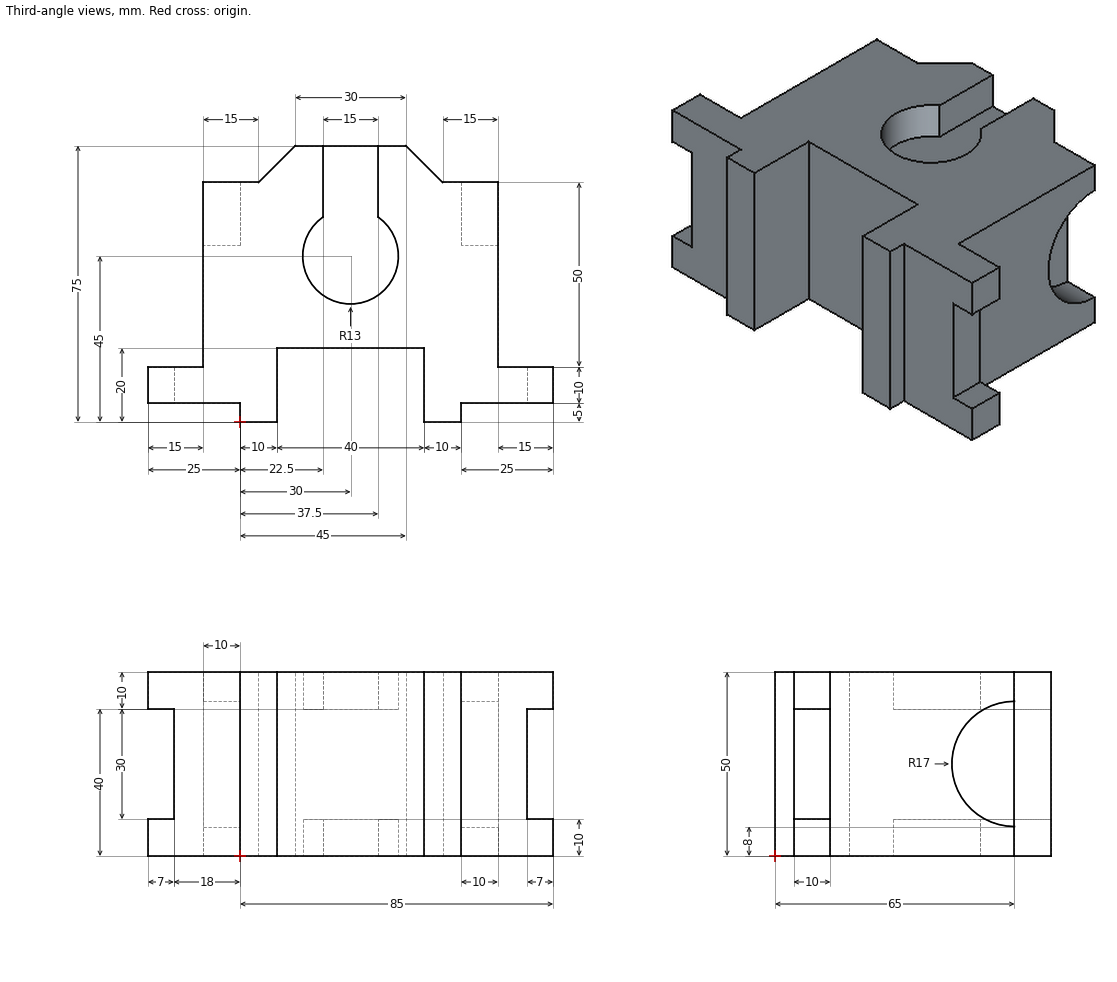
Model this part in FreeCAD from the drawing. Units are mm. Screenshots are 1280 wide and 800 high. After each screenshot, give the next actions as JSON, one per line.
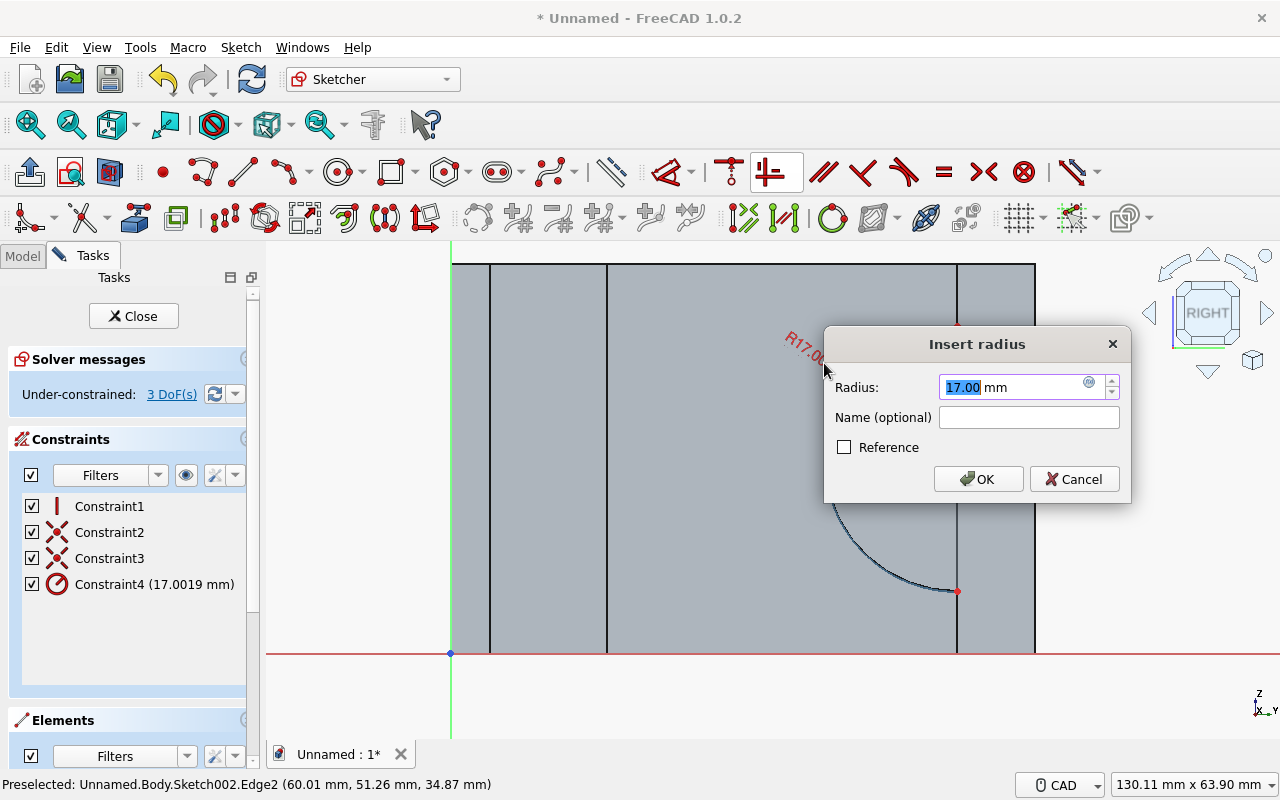
{"action": "type", "text": "17"}
{"action": "key", "text": "Return"}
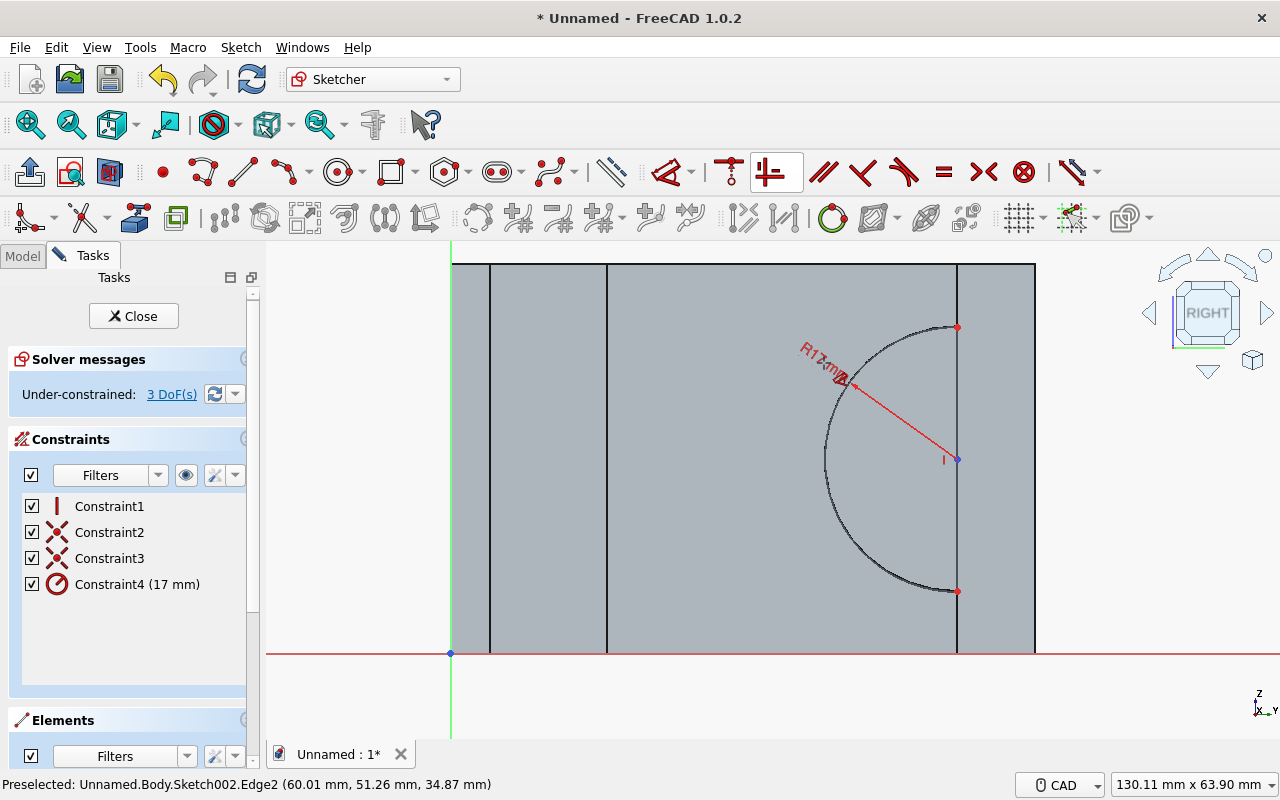
{"action": "left_click", "coordinate": [957, 592]}
{"action": "left_click", "coordinate": [417, 623]}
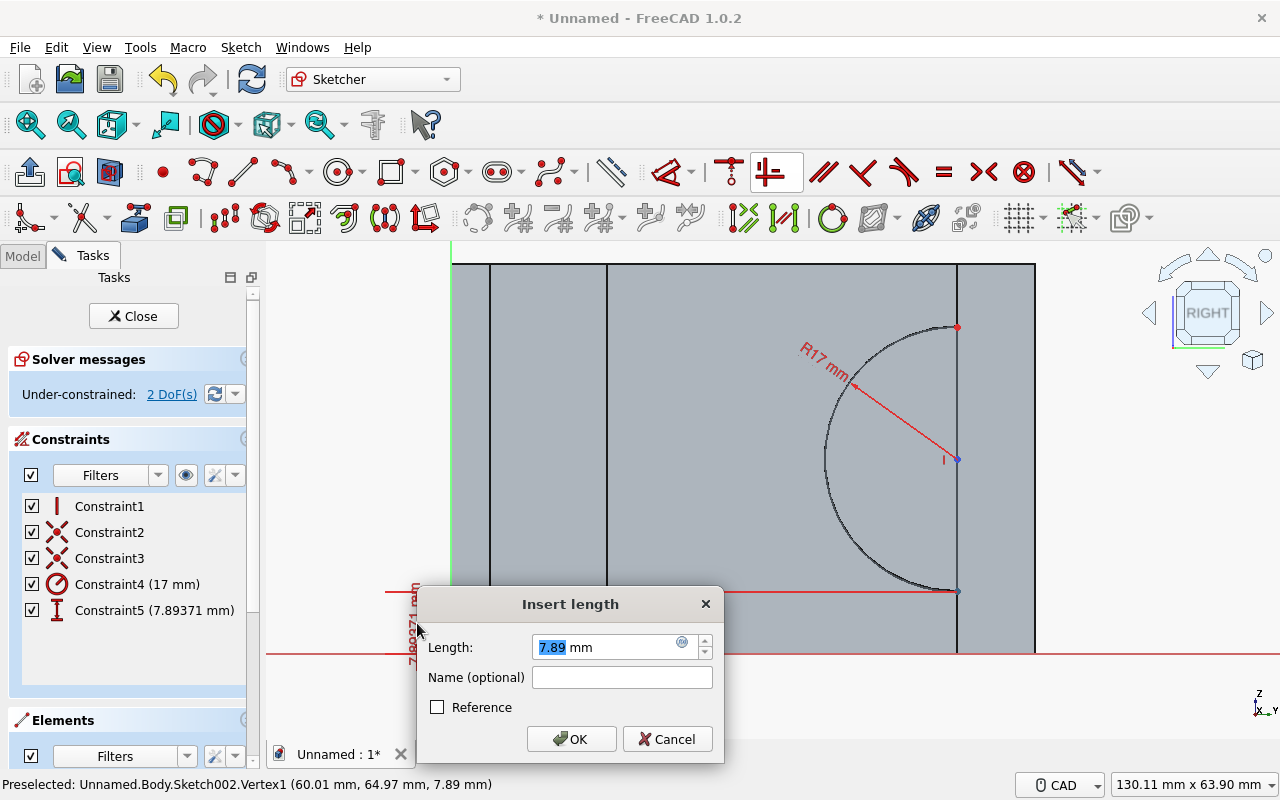
{"action": "type", "text": "8"}
{"action": "key", "text": "Return"}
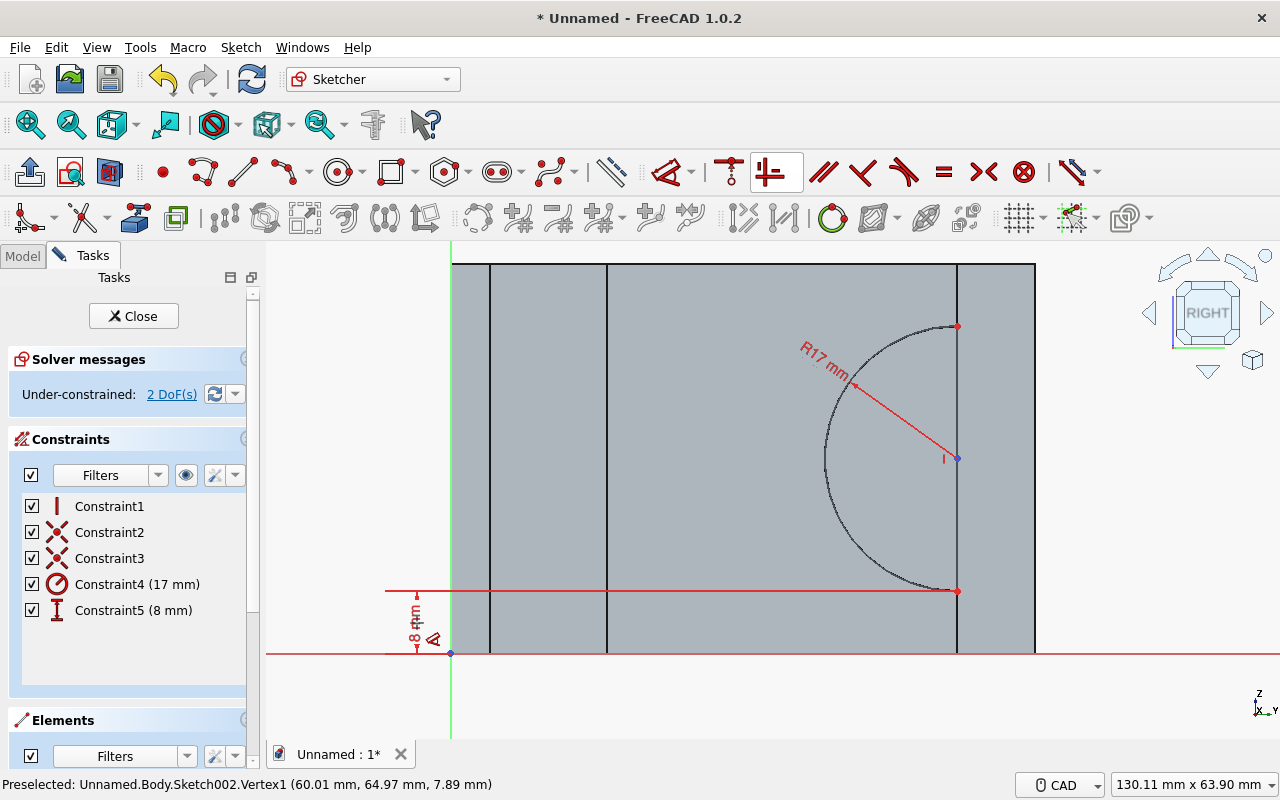
{"action": "left_click", "coordinate": [957, 591]}
{"action": "left_click", "coordinate": [704, 688]}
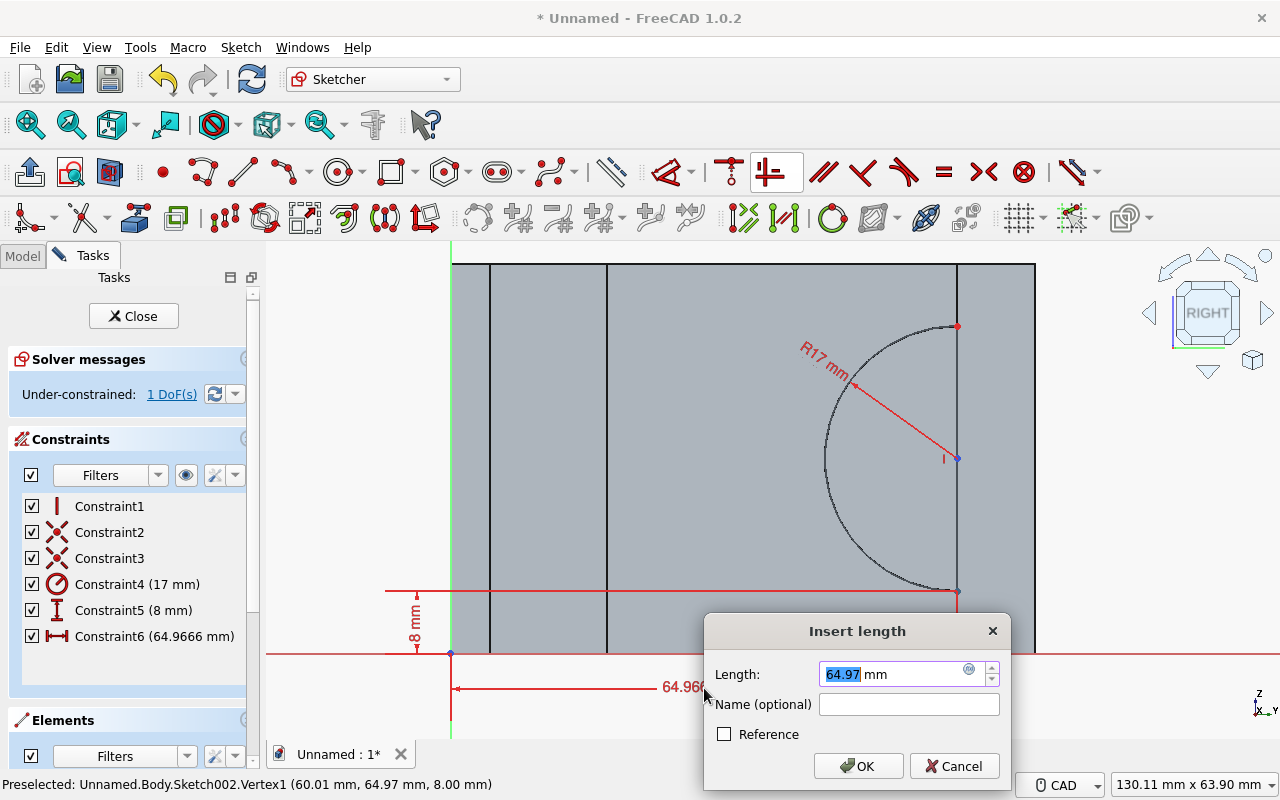
{"action": "type", "text": "65"}
{"action": "key", "text": "Return"}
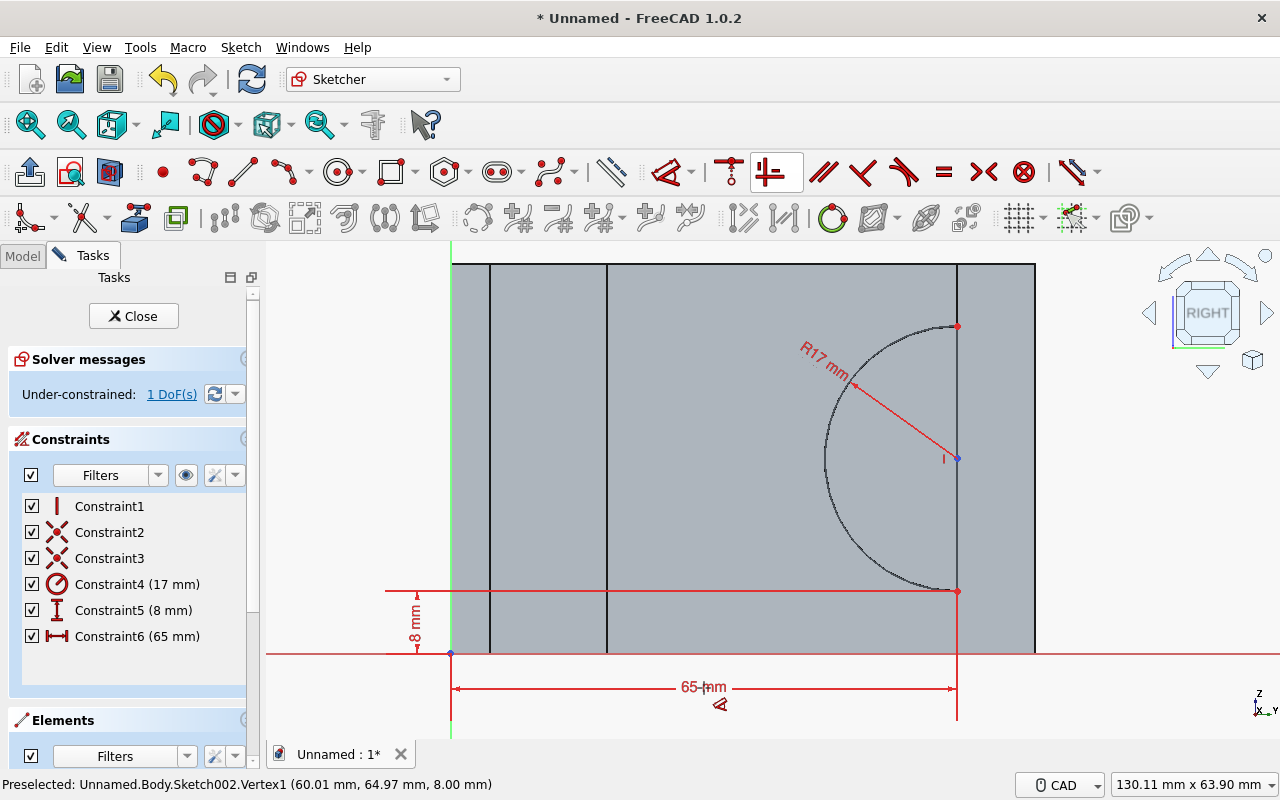
{"action": "left_click", "coordinate": [957, 459]}
{"action": "left_click", "coordinate": [588, 688]}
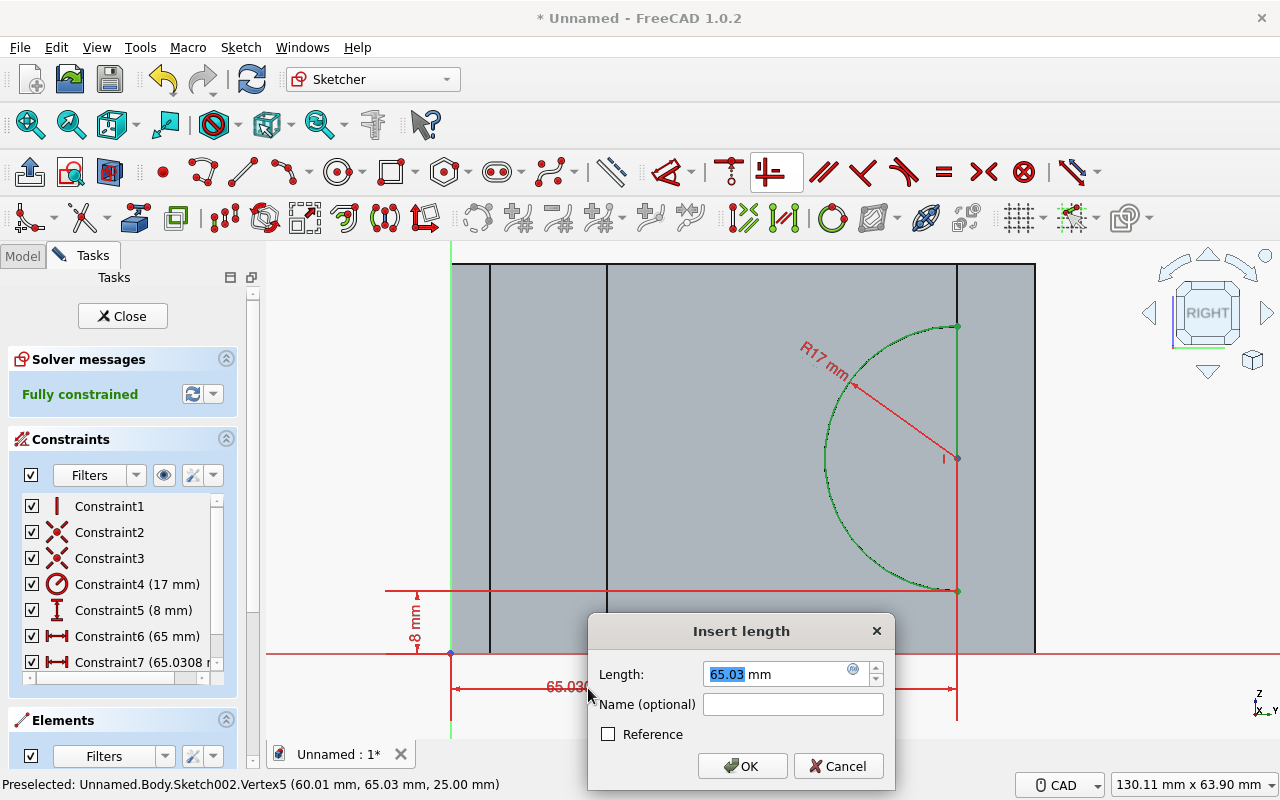
{"action": "type", "text": "65"}
{"action": "key", "text": "Return"}
{"action": "key", "text": "Escape"}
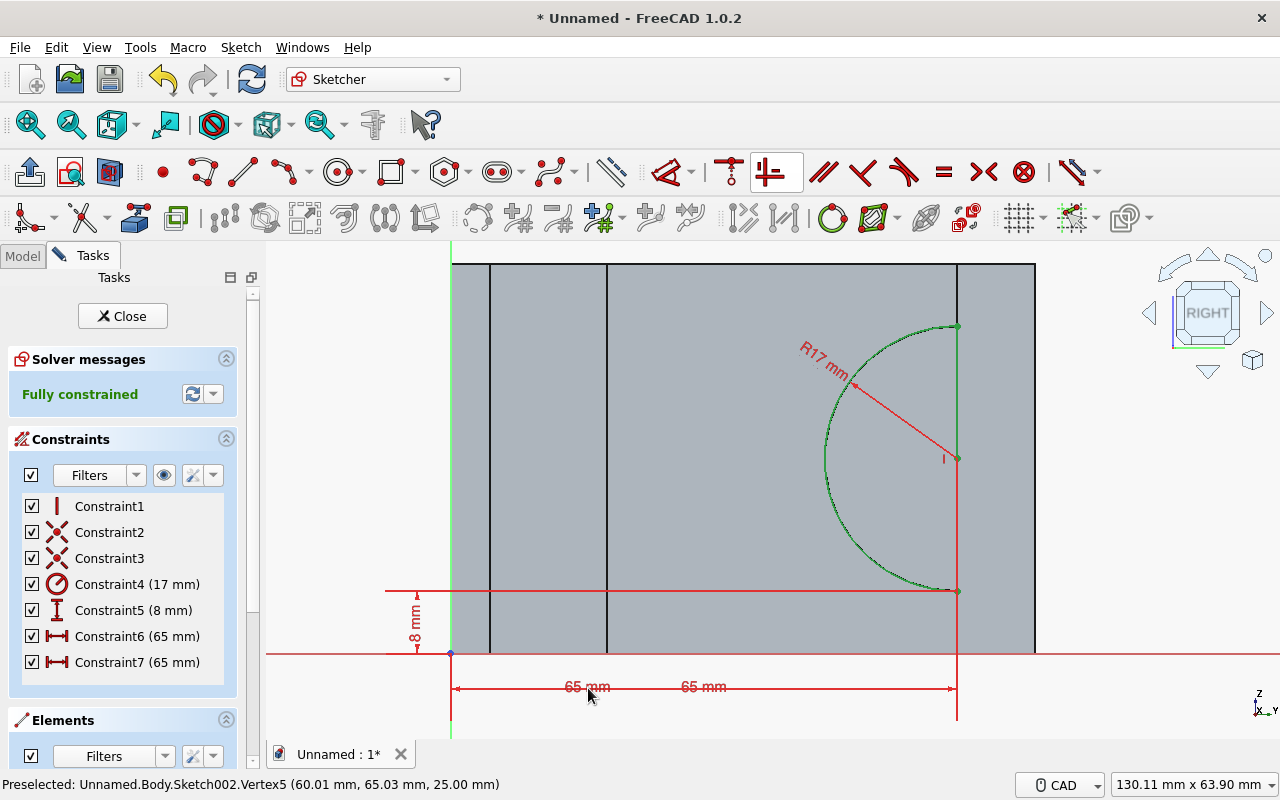
{"action": "left_click", "coordinate": [123, 316]}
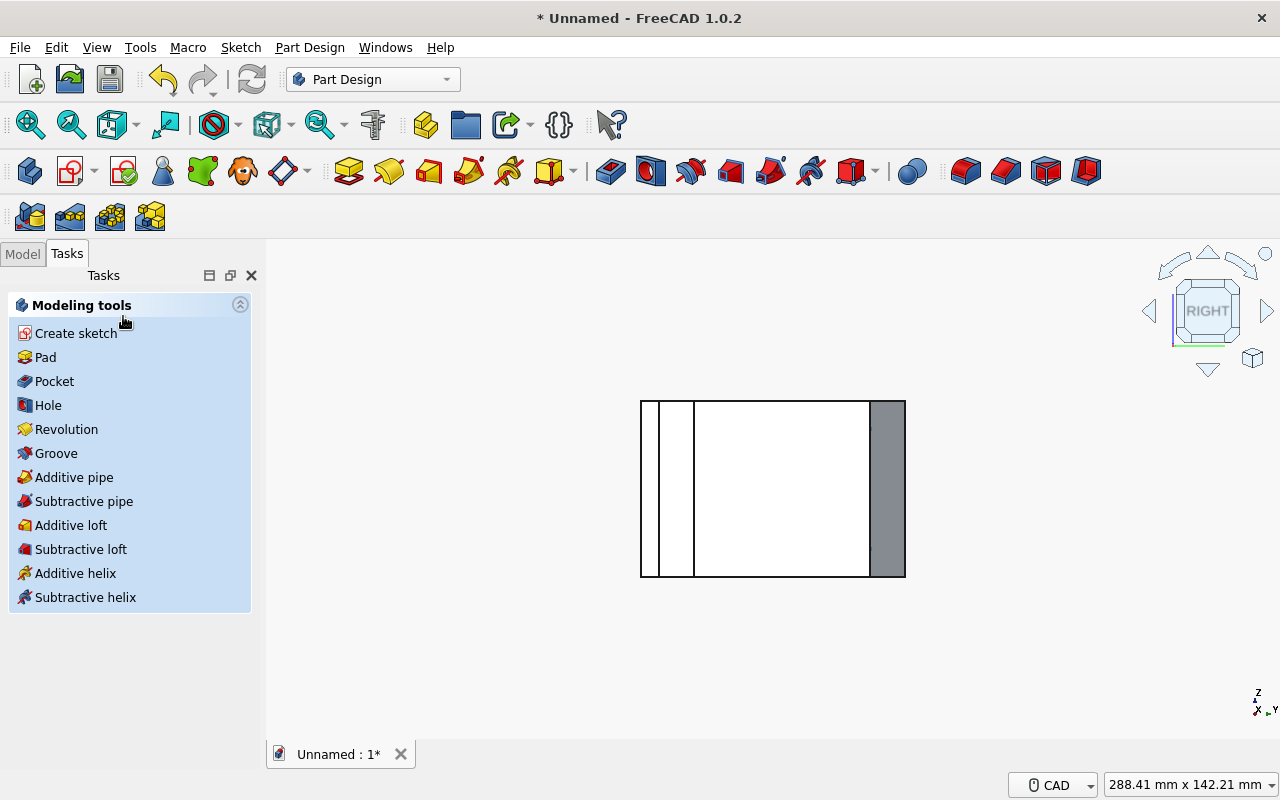
{"action": "left_click", "coordinate": [612, 172]}